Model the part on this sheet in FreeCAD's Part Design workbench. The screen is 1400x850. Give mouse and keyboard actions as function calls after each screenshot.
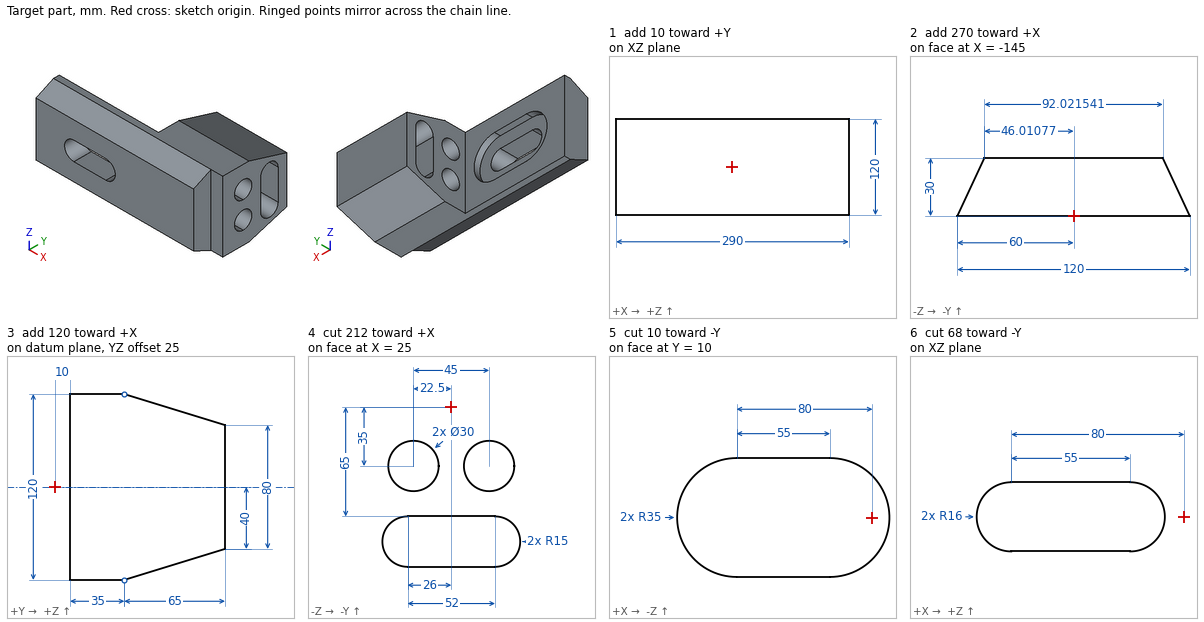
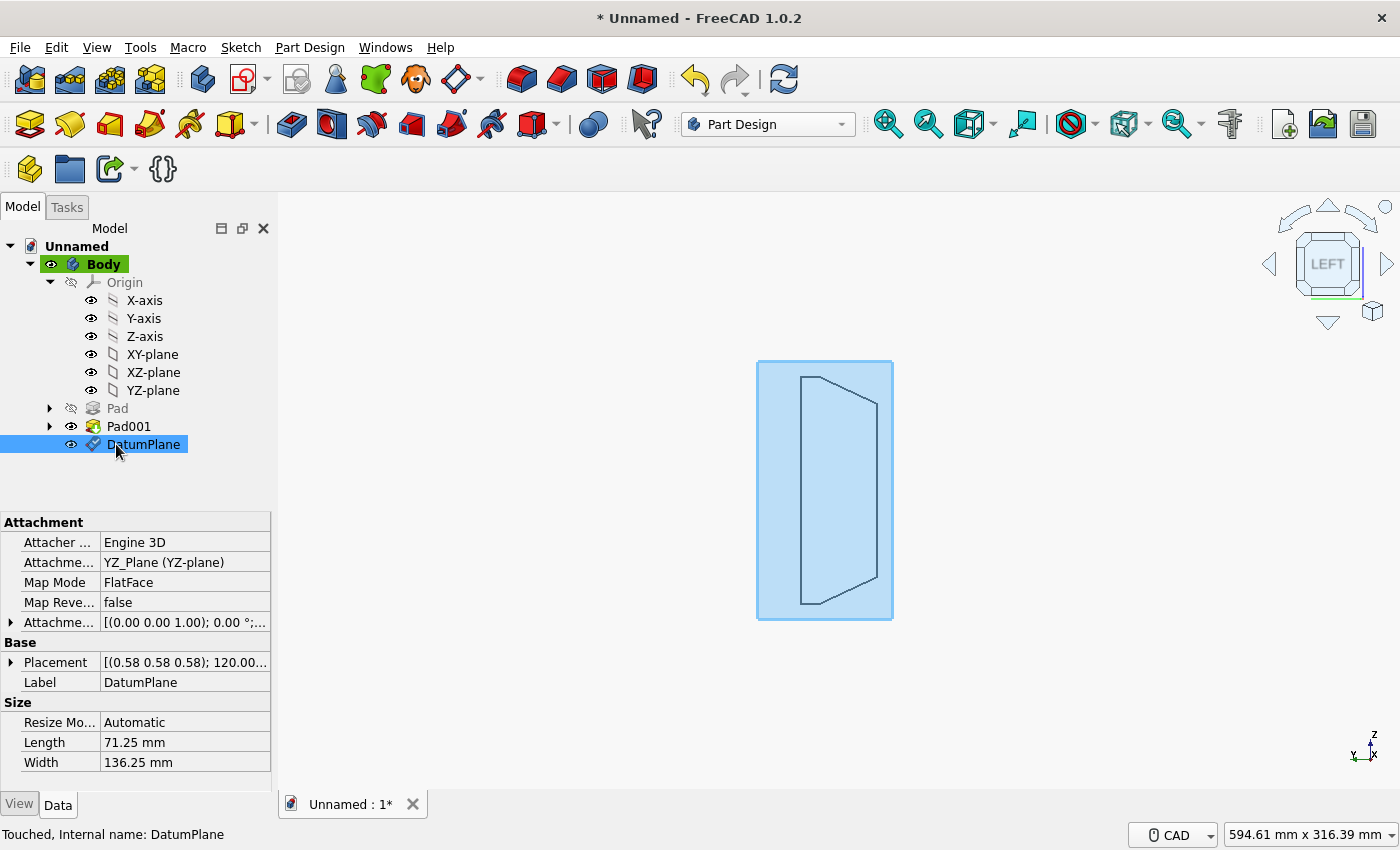
click(244, 80)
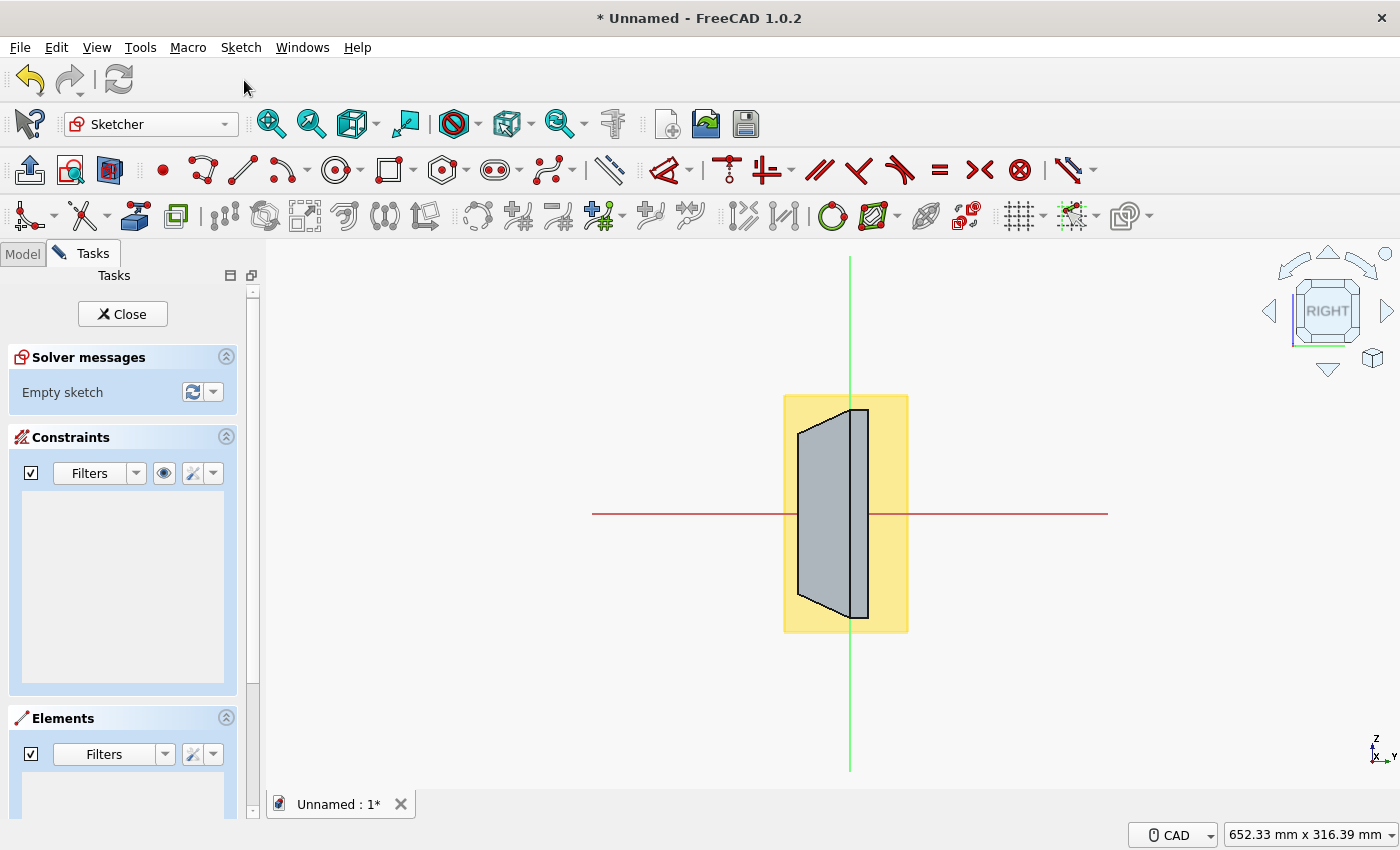
key(q)
key(s)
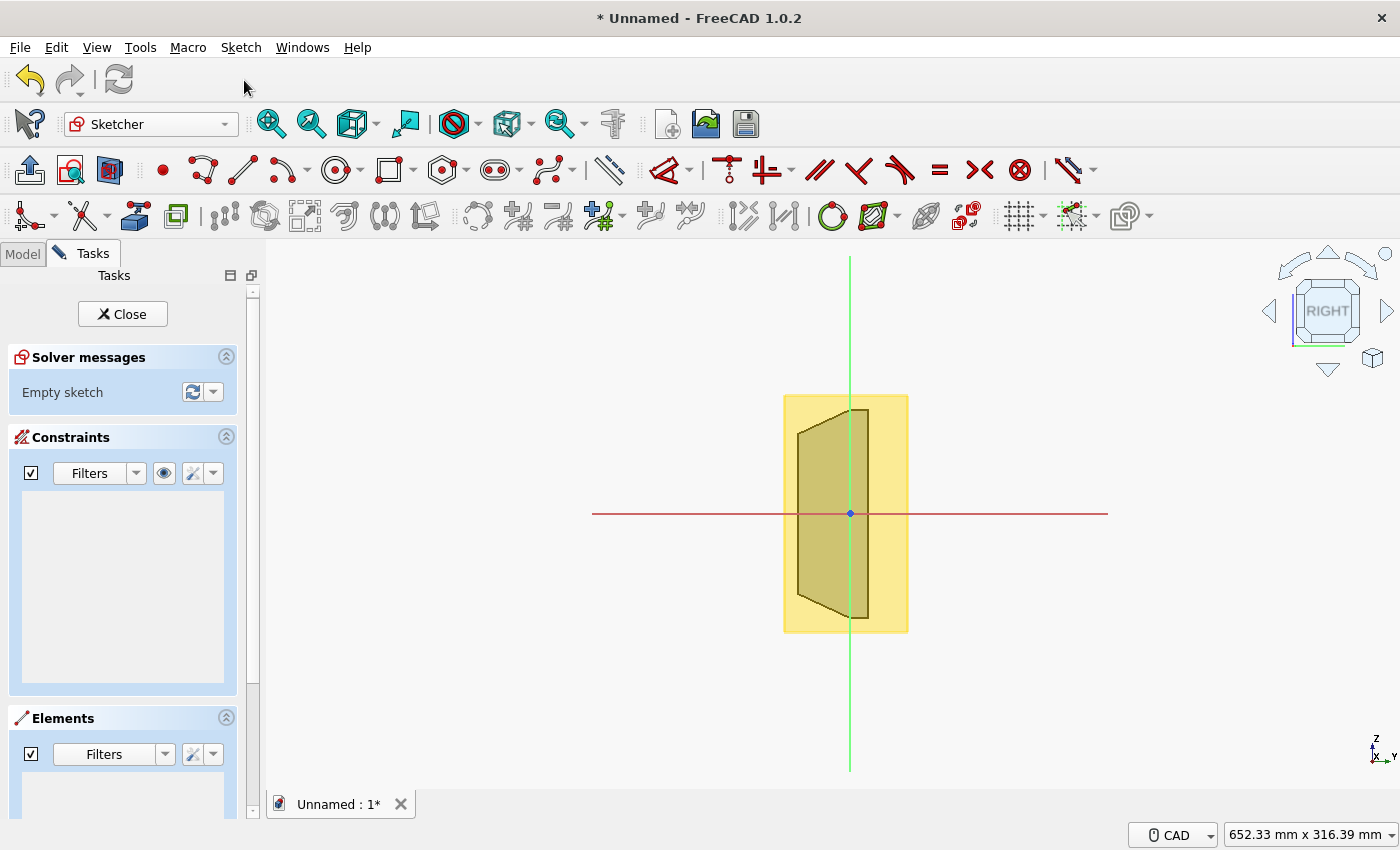
scroll(1167, 514, up, 3)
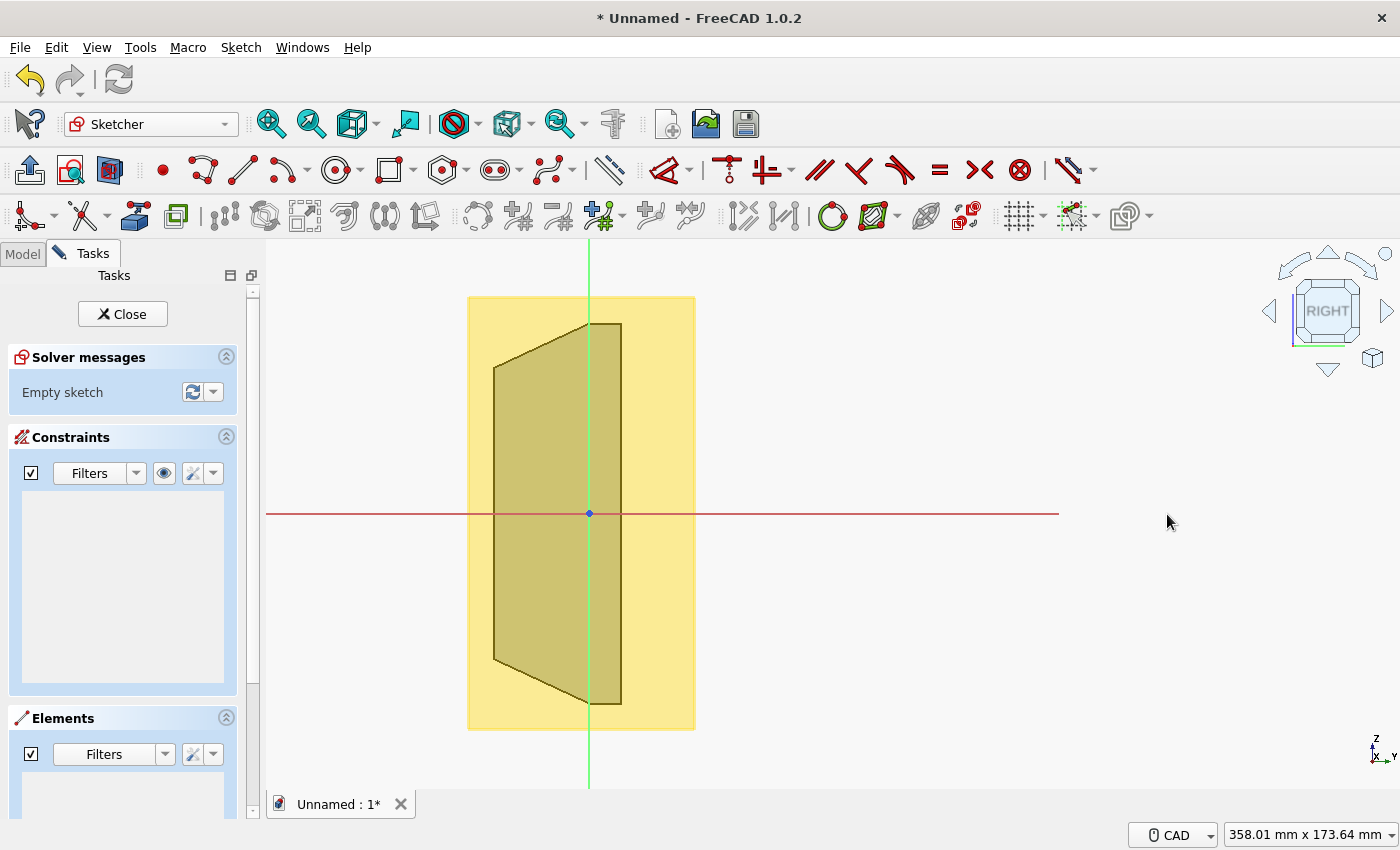
key(g)
key(m)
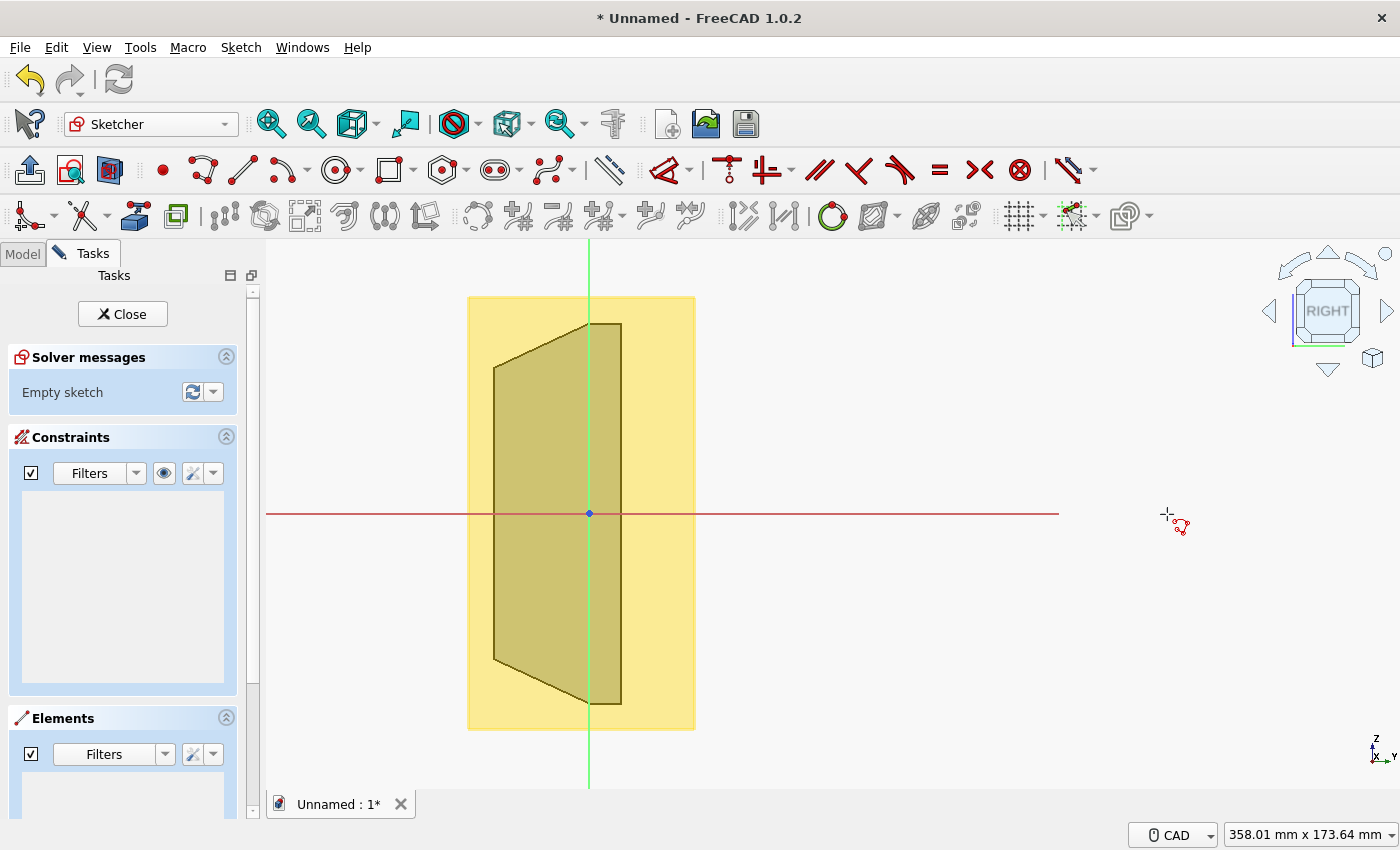
click(621, 324)
click(621, 704)
click(732, 704)
click(938, 640)
click(938, 387)
click(732, 324)
click(621, 325)
key(Escape)
key(Escape)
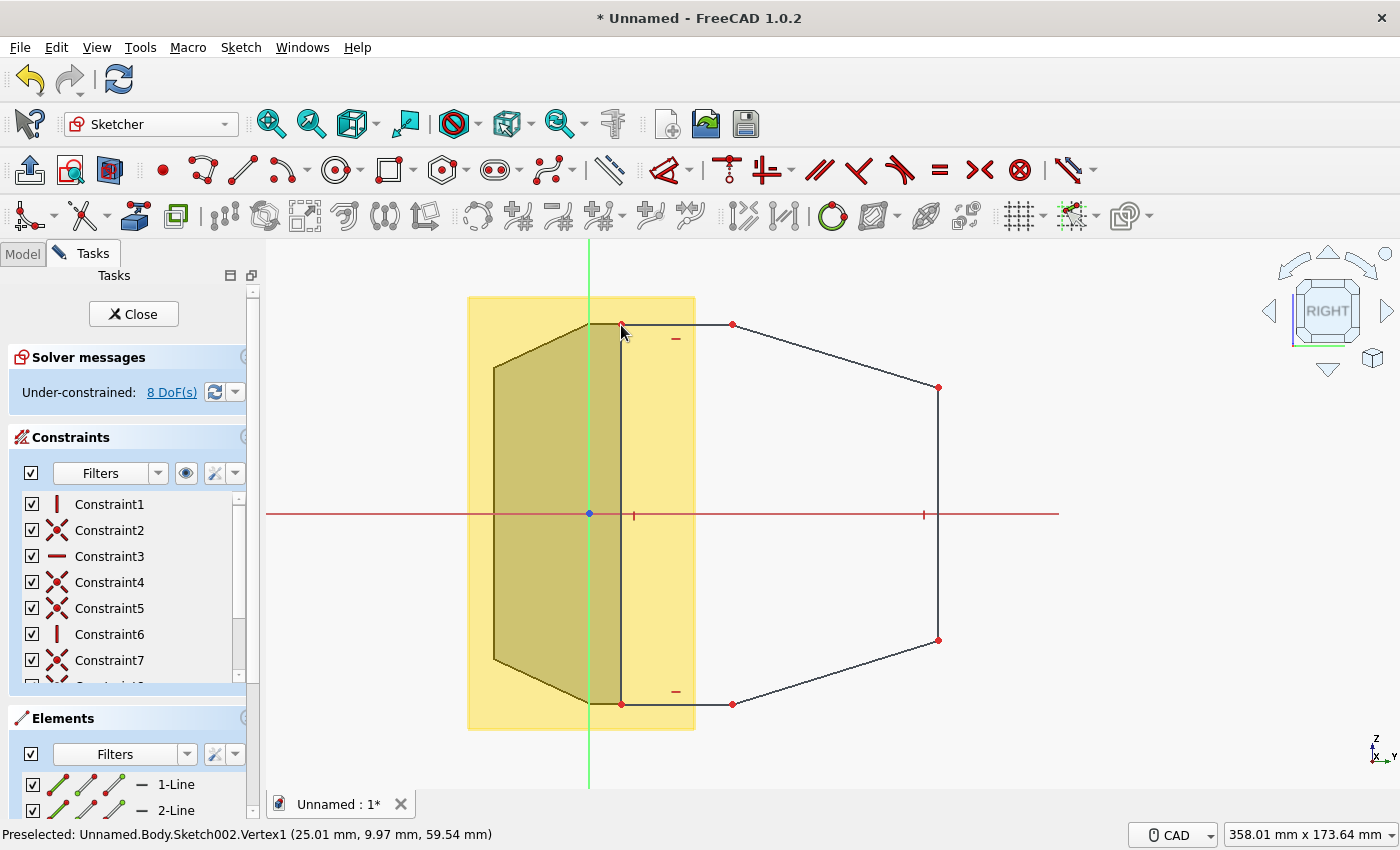
click(732, 705)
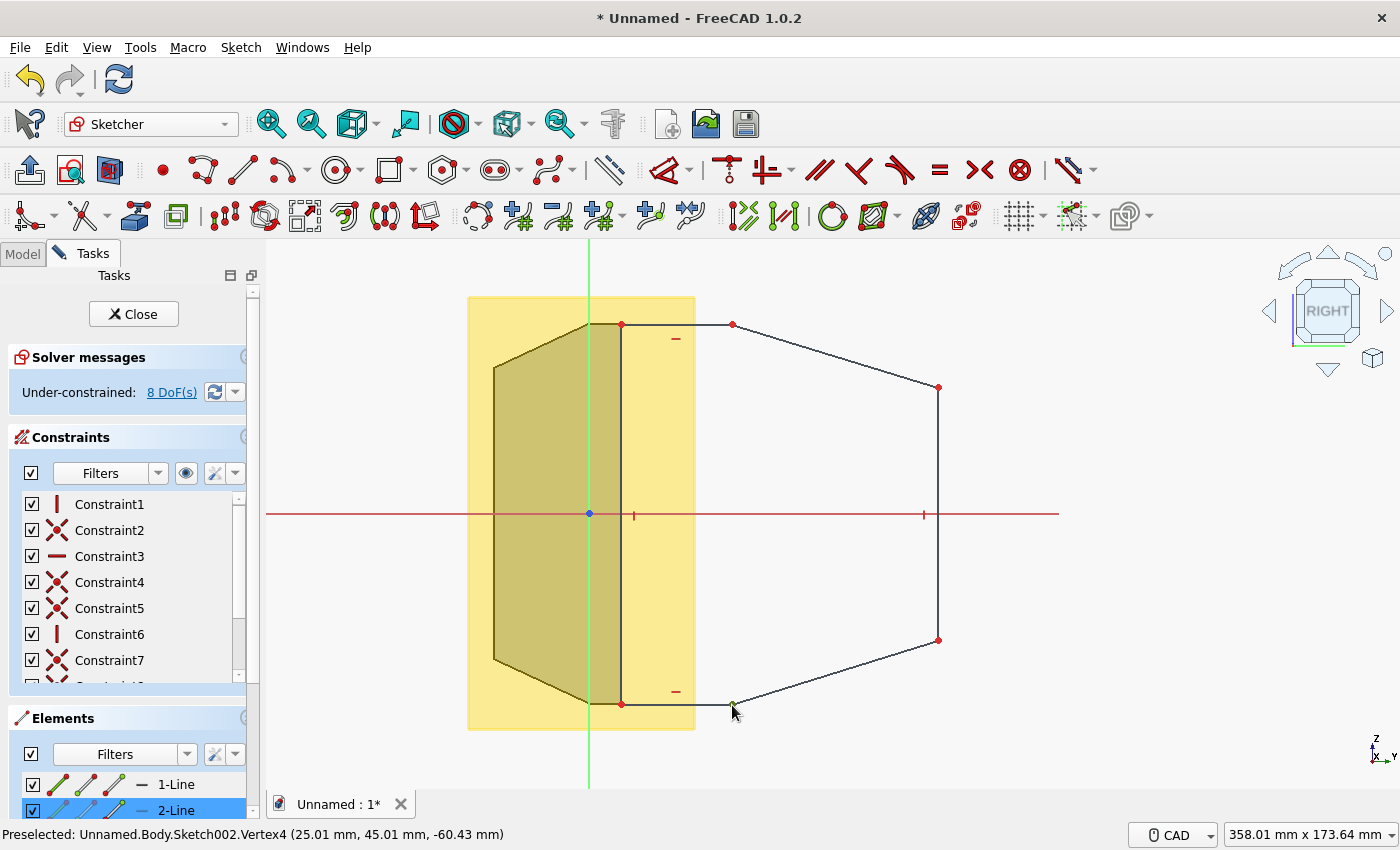
click(732, 325)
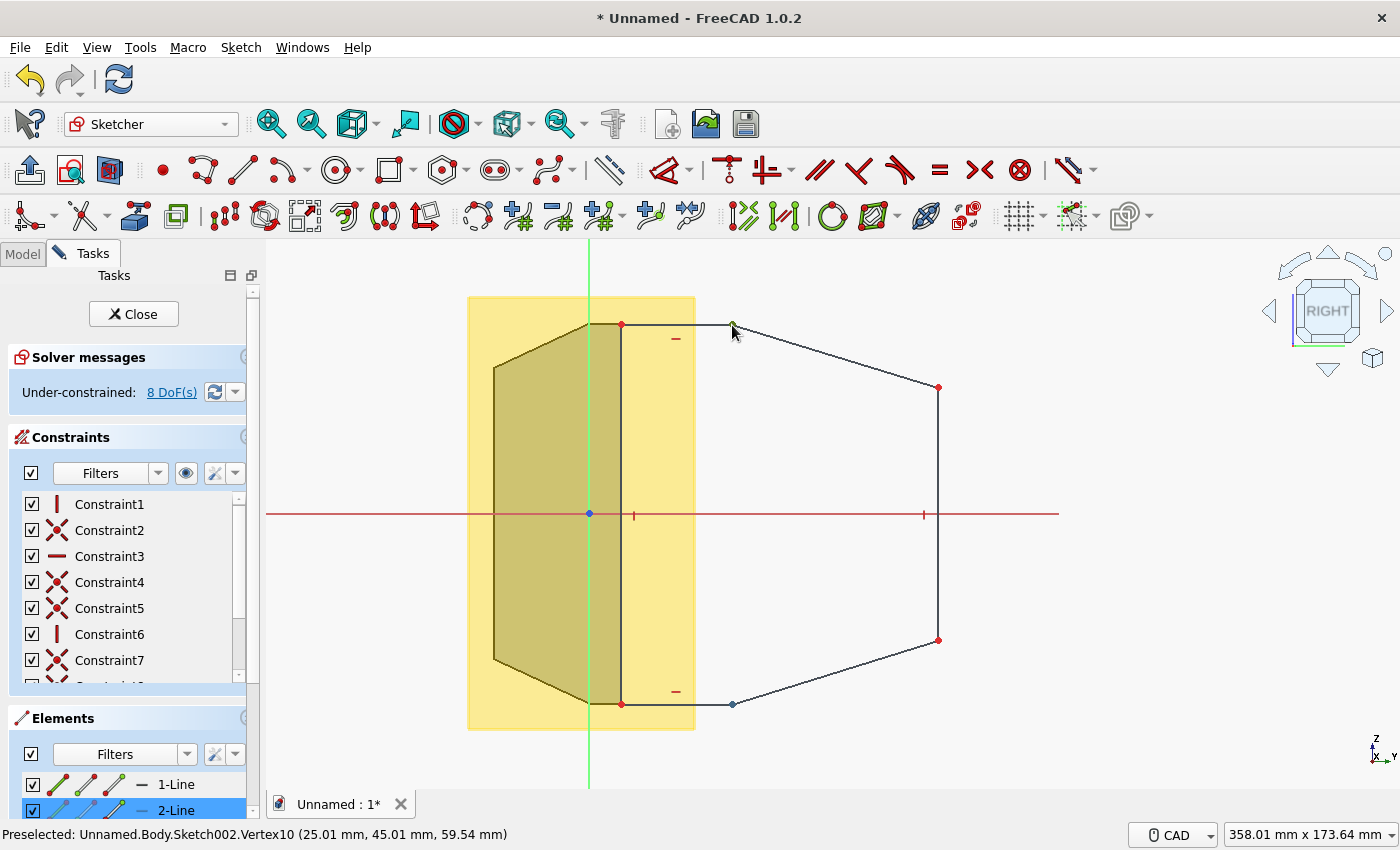
click(361, 514)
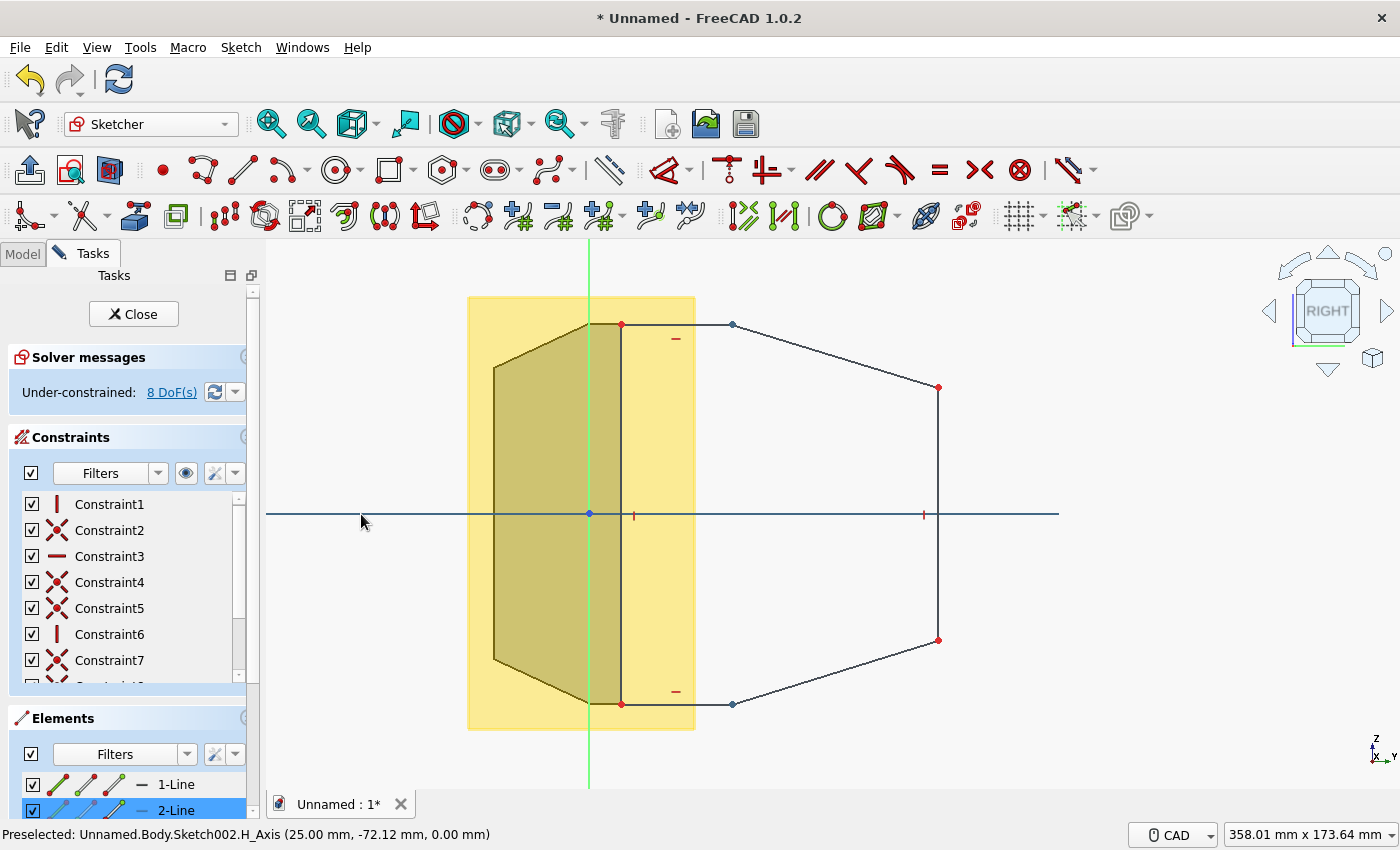
click(980, 170)